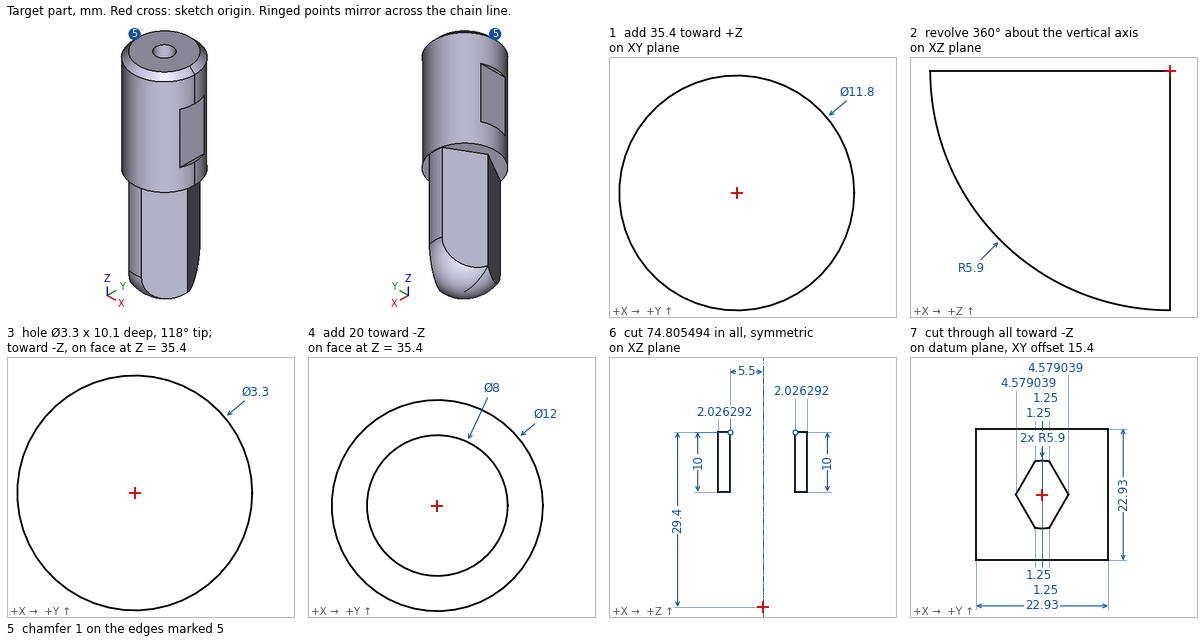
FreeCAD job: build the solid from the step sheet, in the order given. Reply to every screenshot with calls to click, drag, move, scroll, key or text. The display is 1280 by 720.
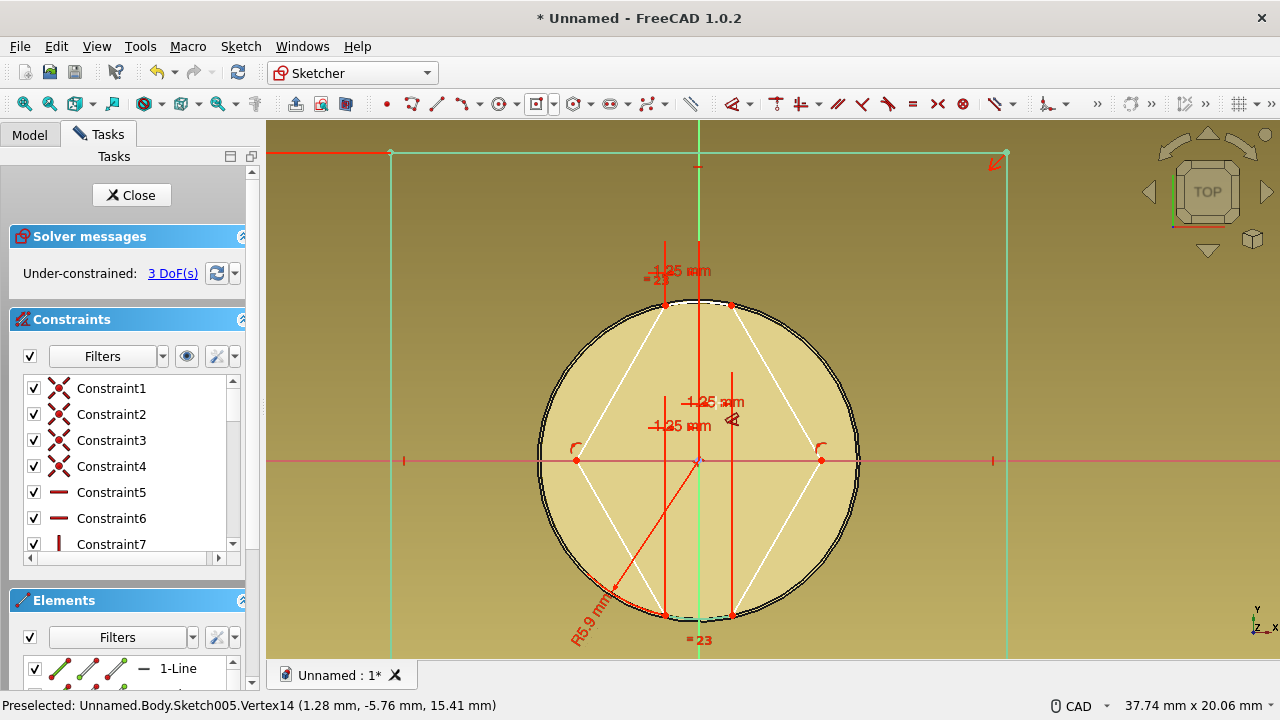
click(732, 306)
click(715, 495)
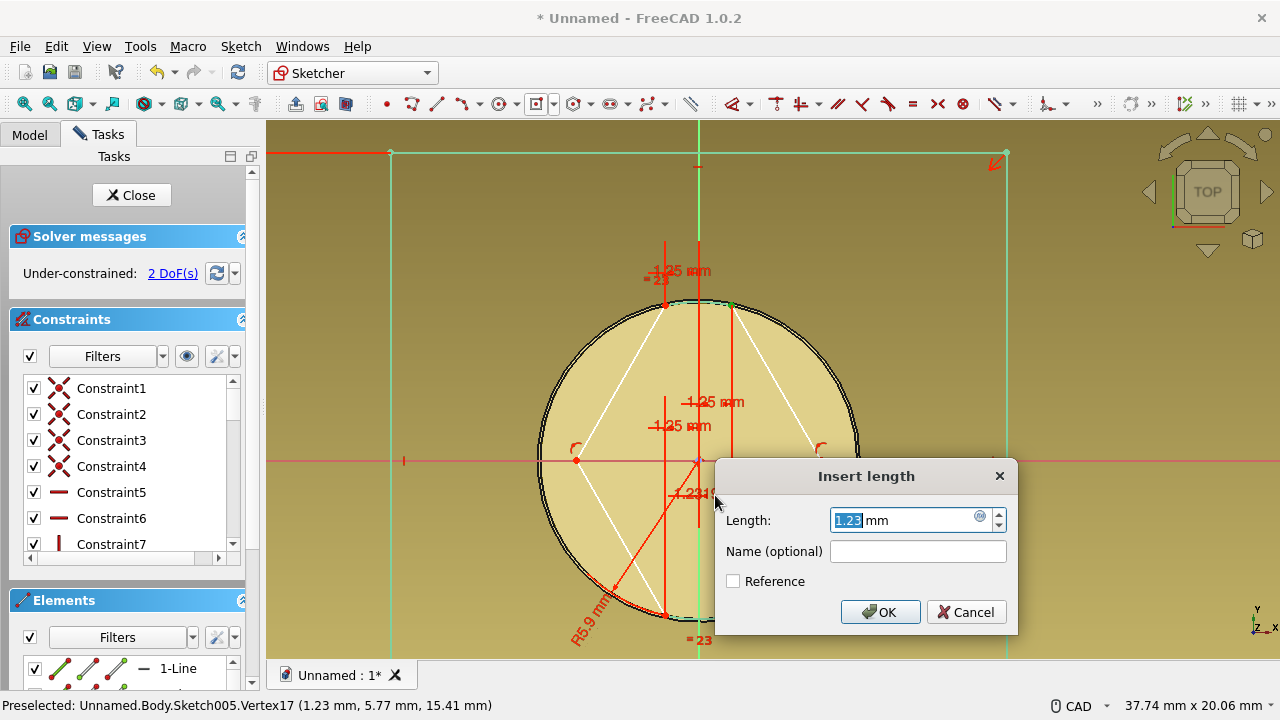
text(1.25)
key(Return)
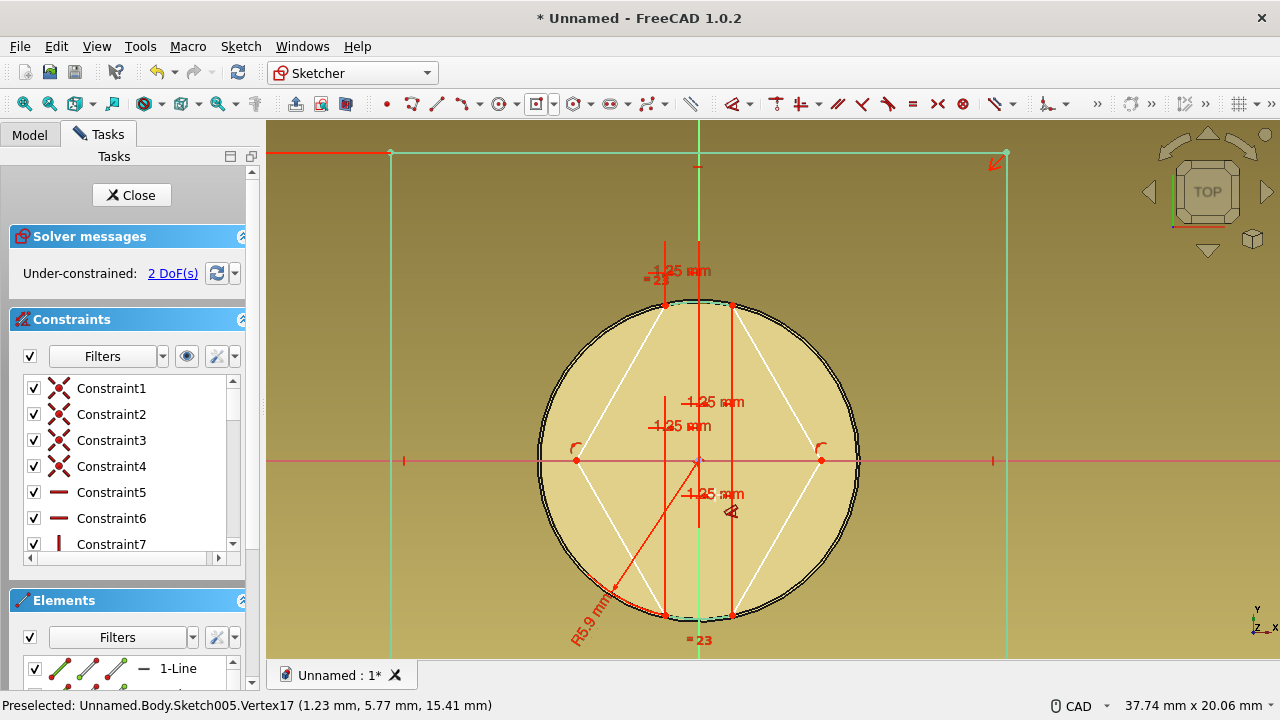
click(577, 461)
click(638, 495)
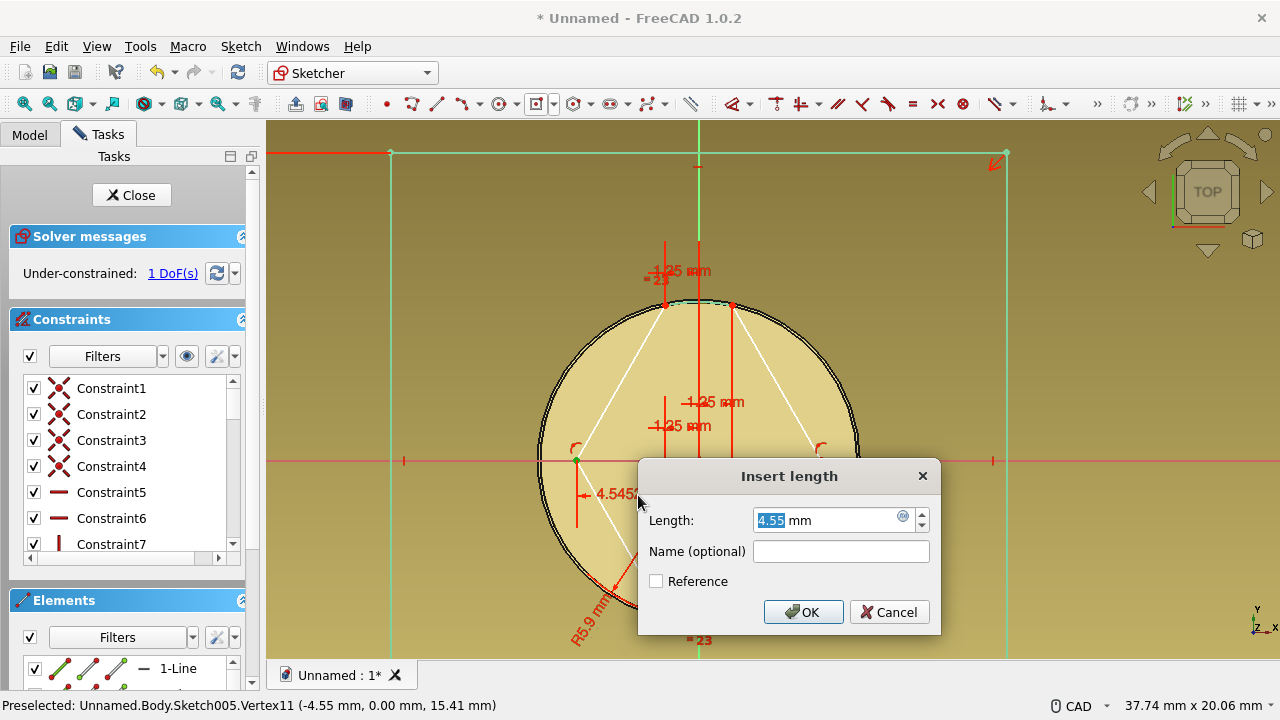
text(4.579039)
key(Return)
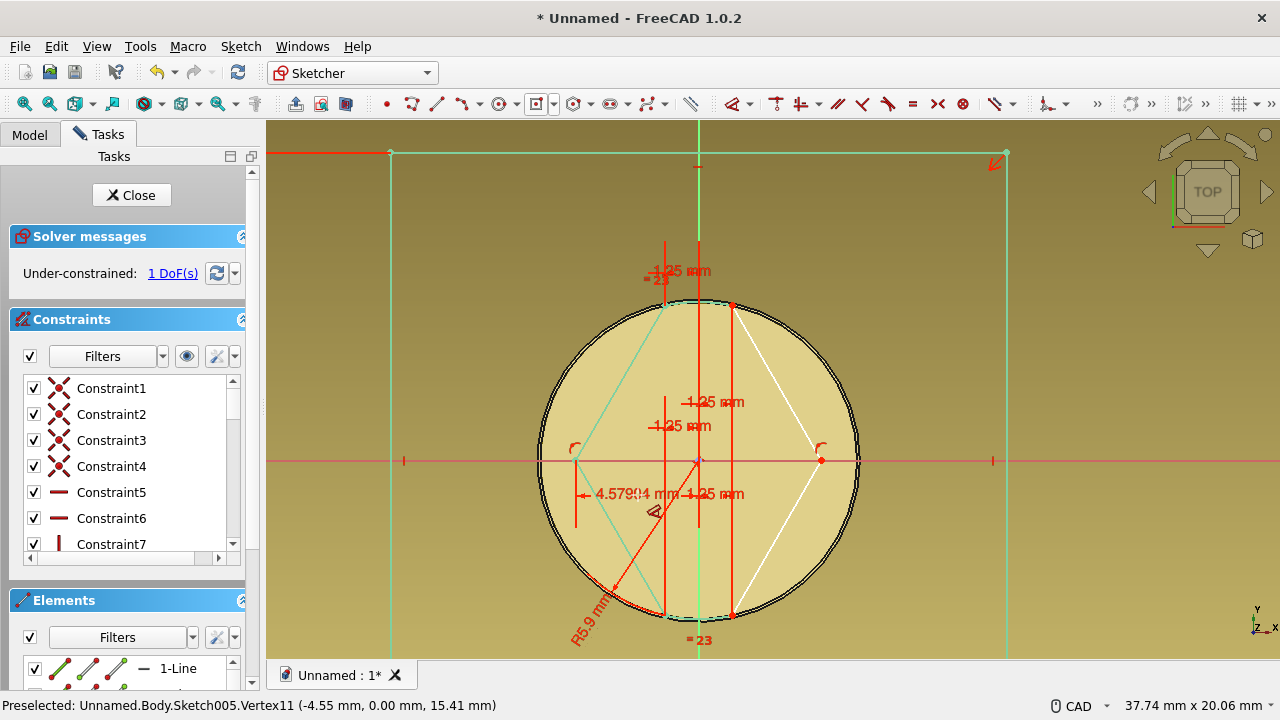
click(821, 461)
click(760, 427)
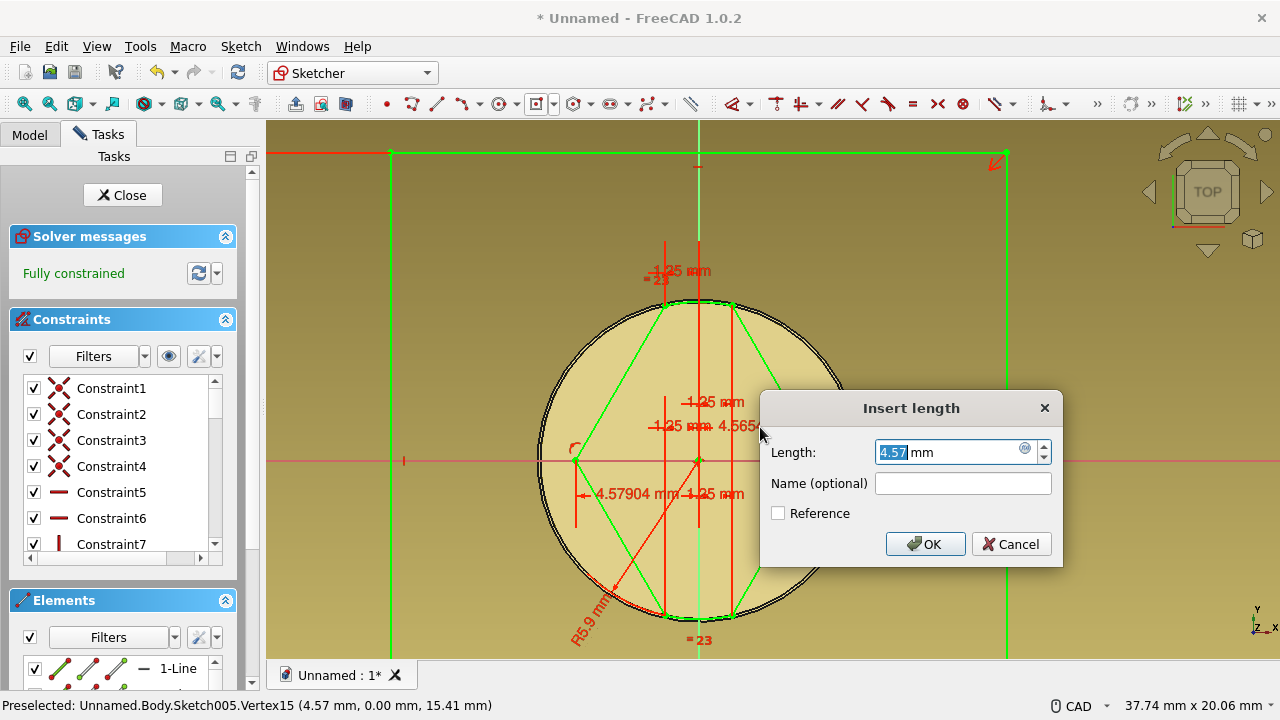
text(4.579039)
key(Return)
key(Escape)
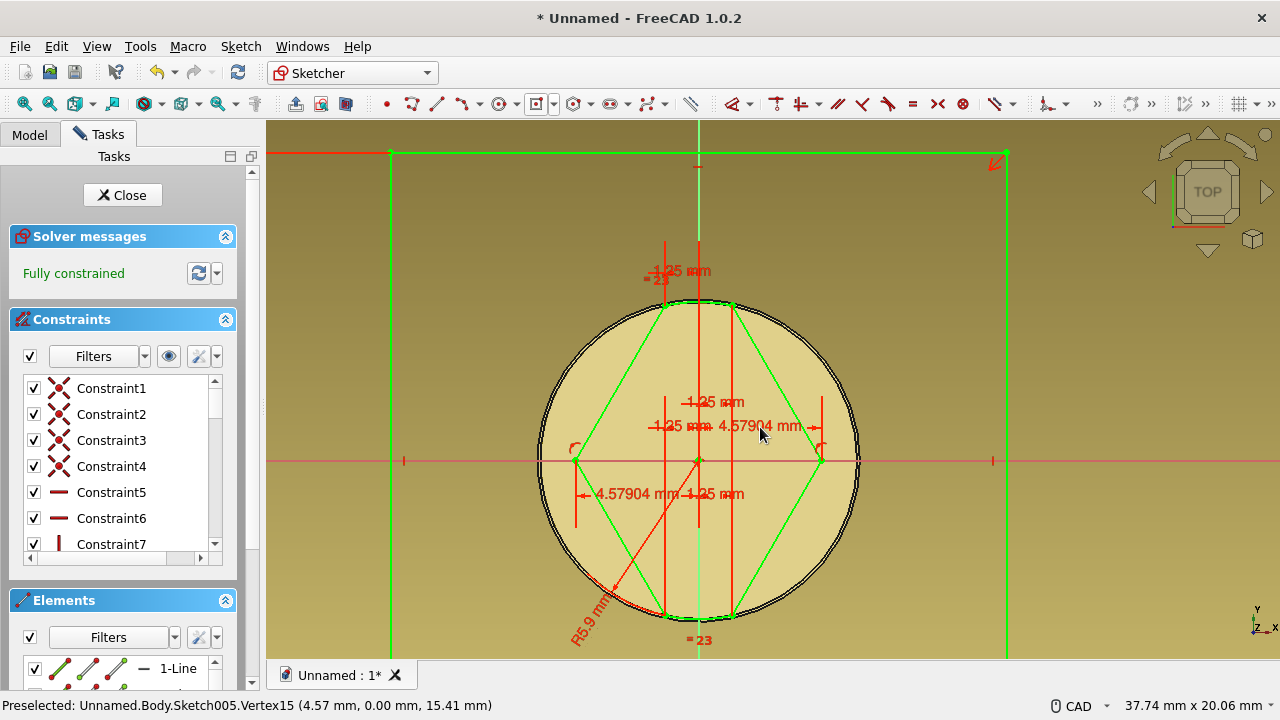
click(123, 195)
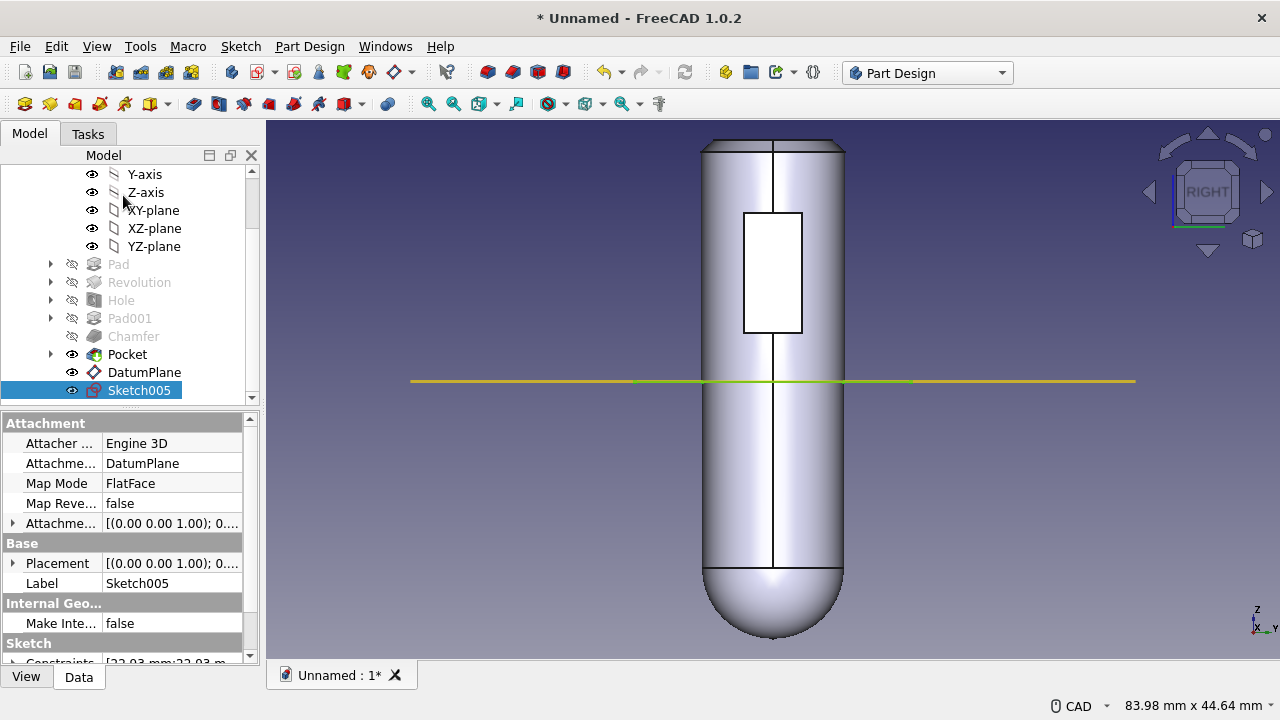
click(194, 104)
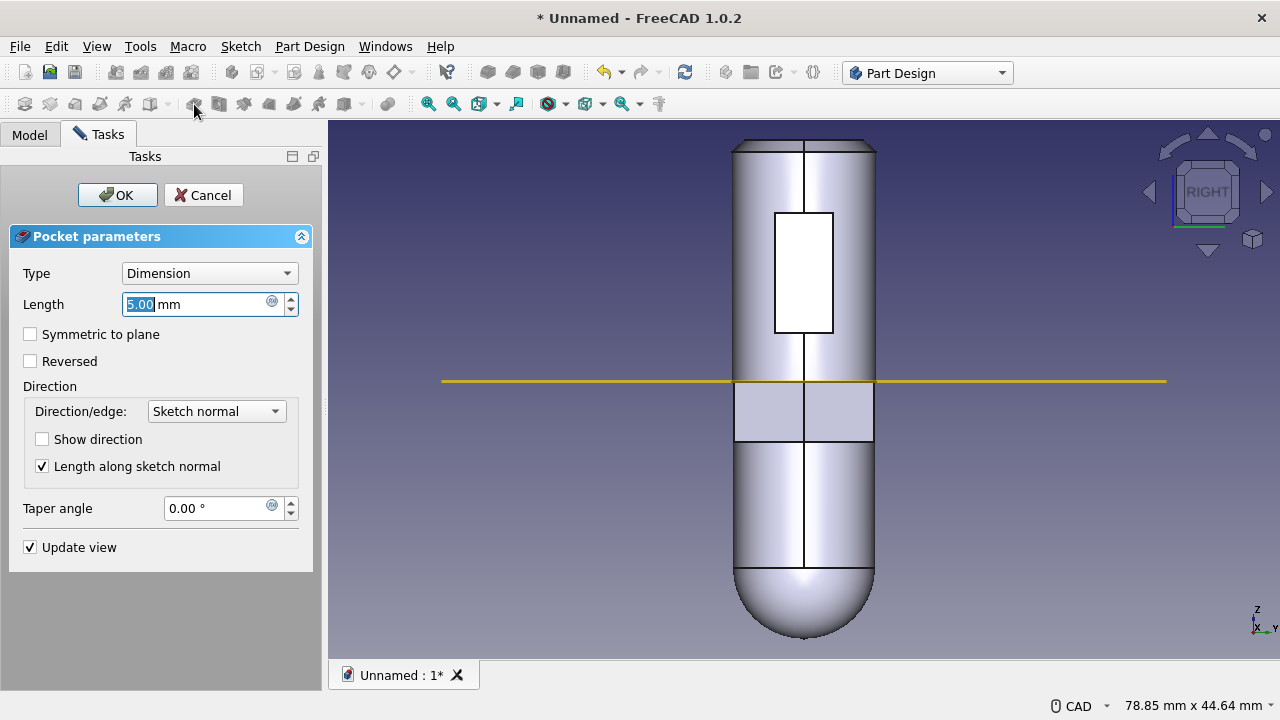
click(210, 274)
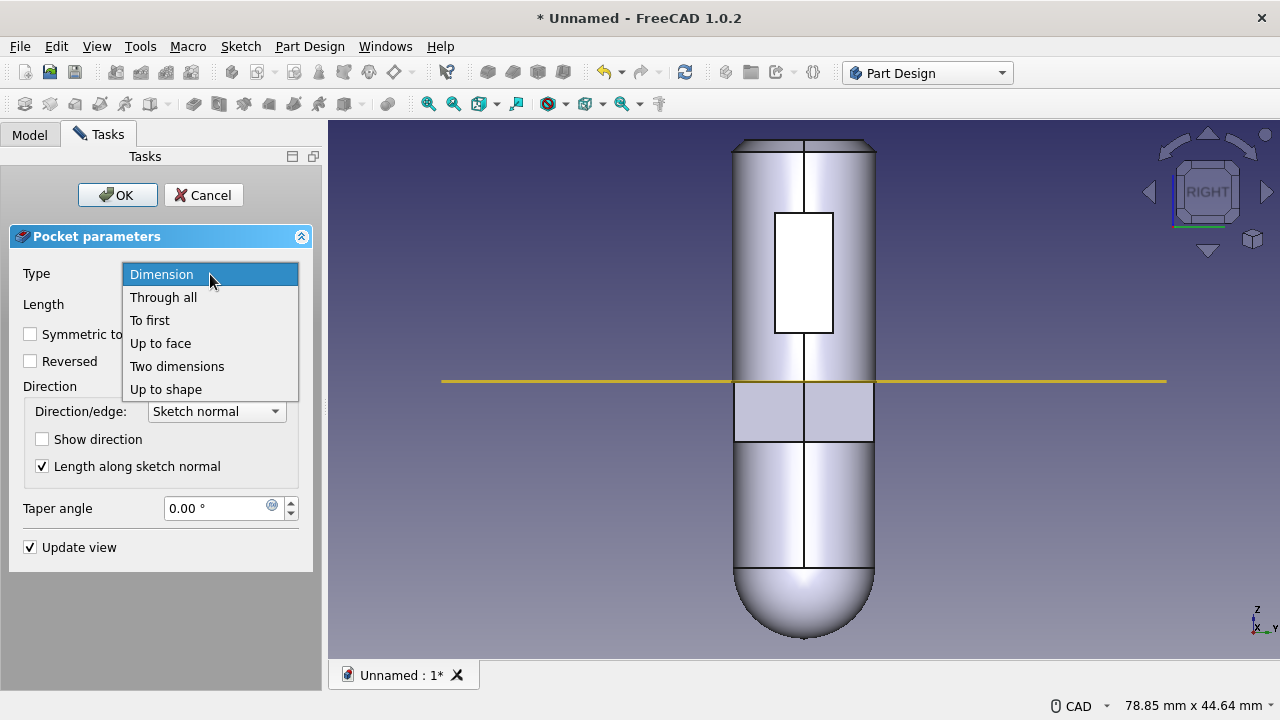
click(208, 298)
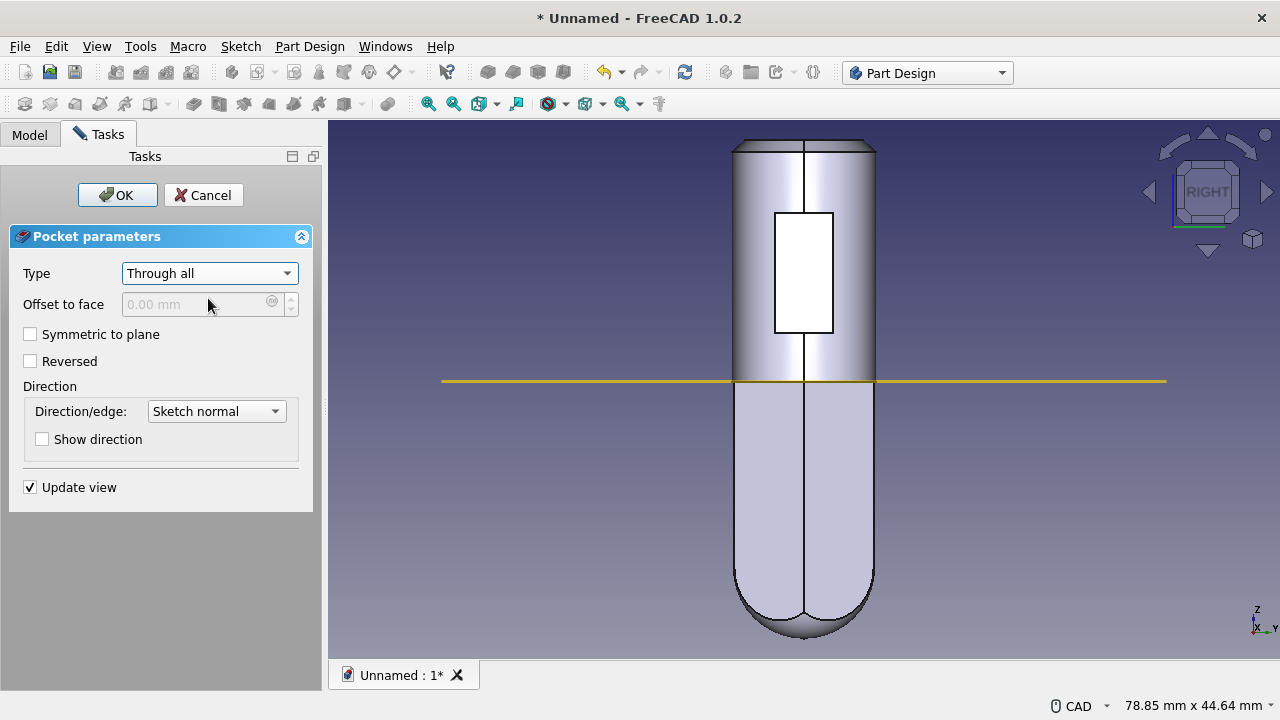
click(118, 195)